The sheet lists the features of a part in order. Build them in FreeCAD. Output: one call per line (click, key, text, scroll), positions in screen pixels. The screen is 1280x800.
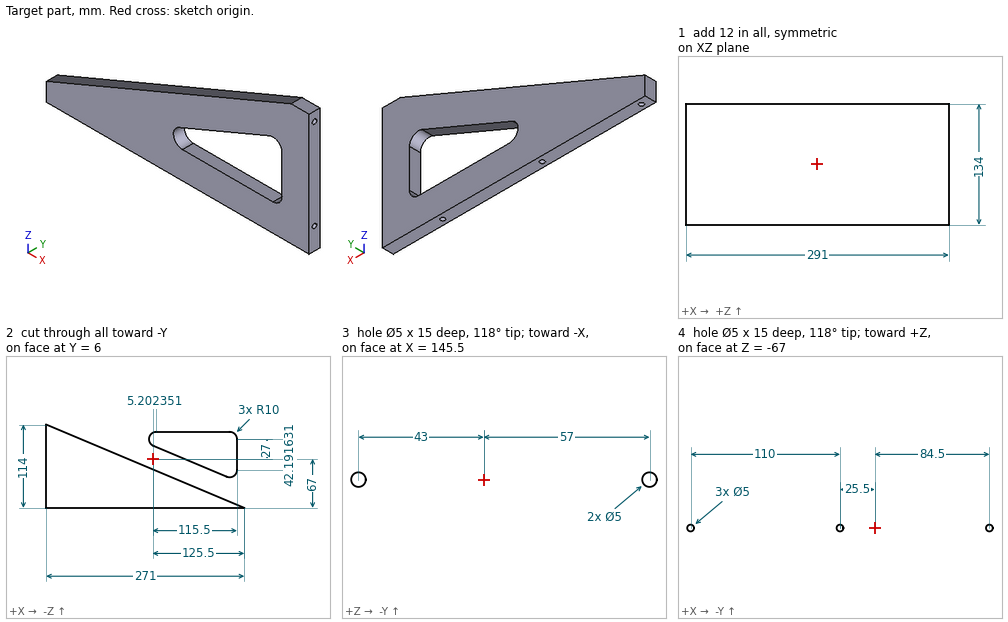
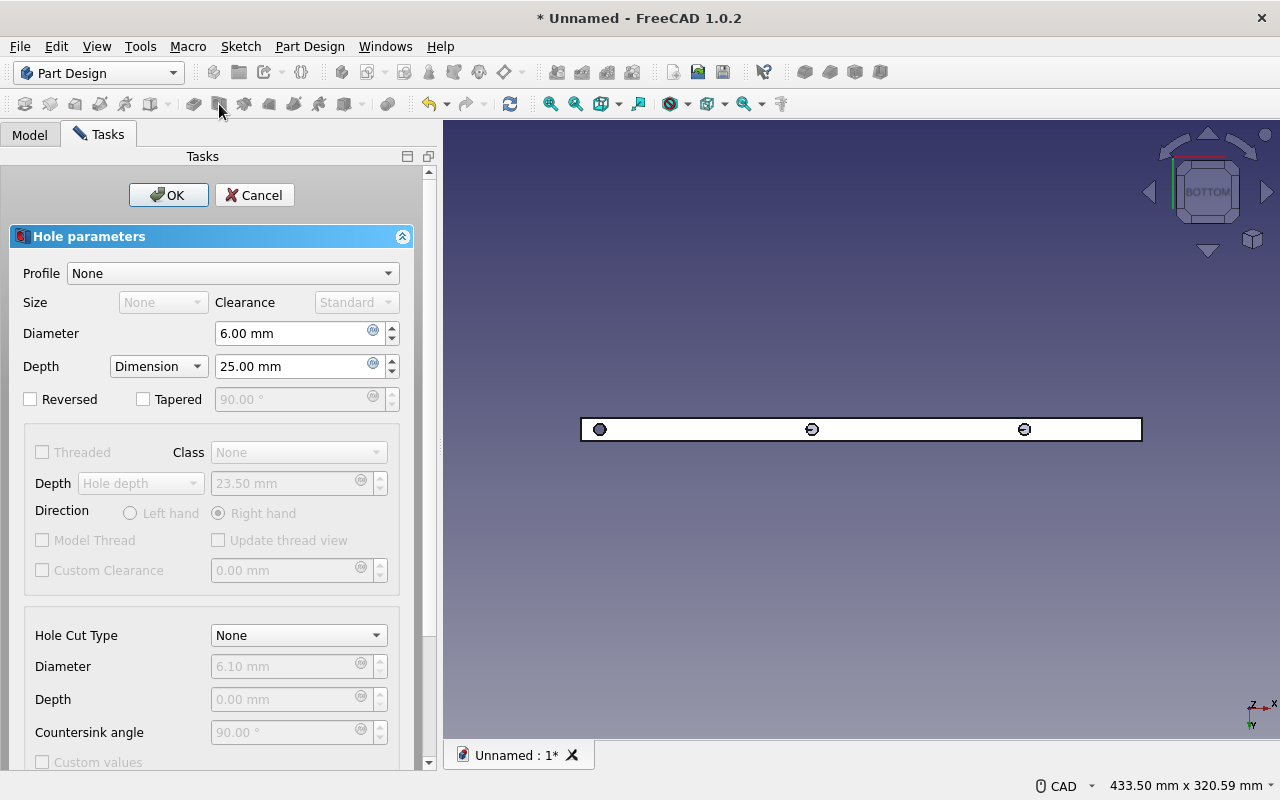
triple_click(300, 334)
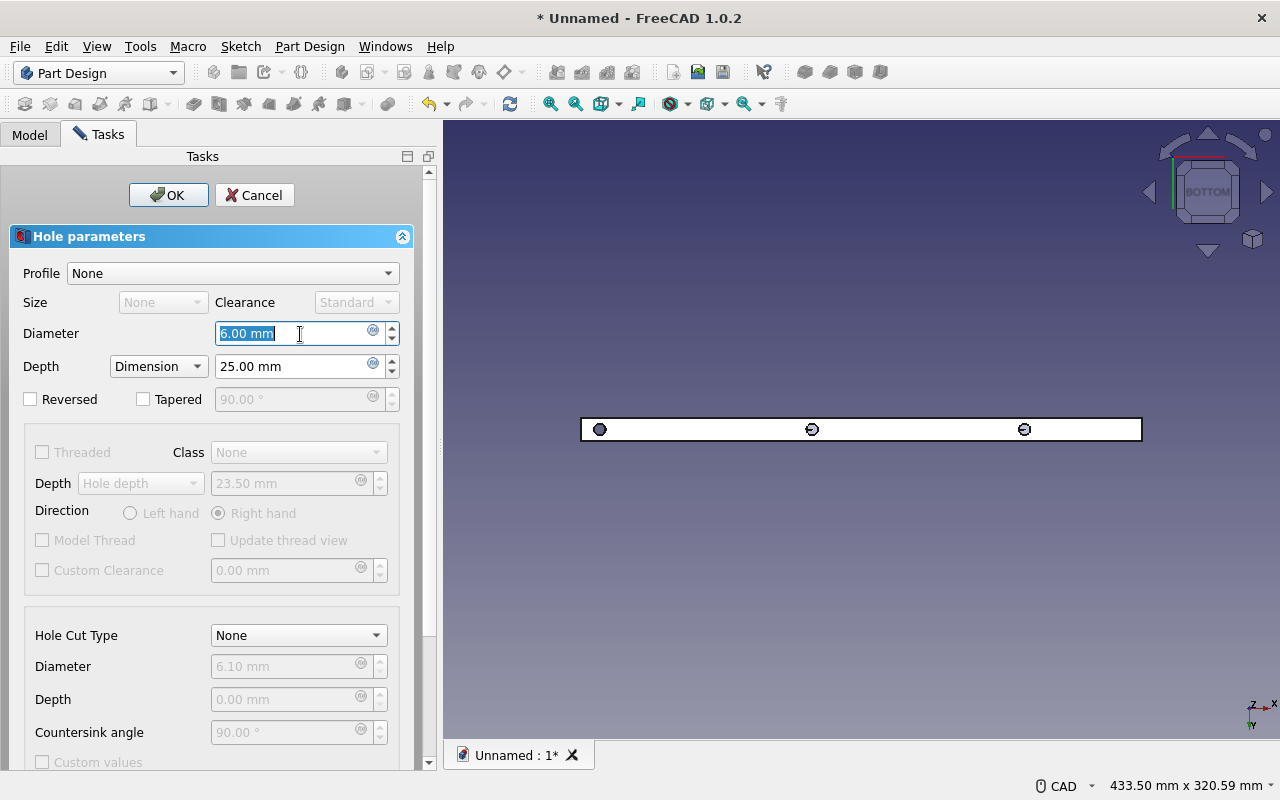
text(5)
key(Tab)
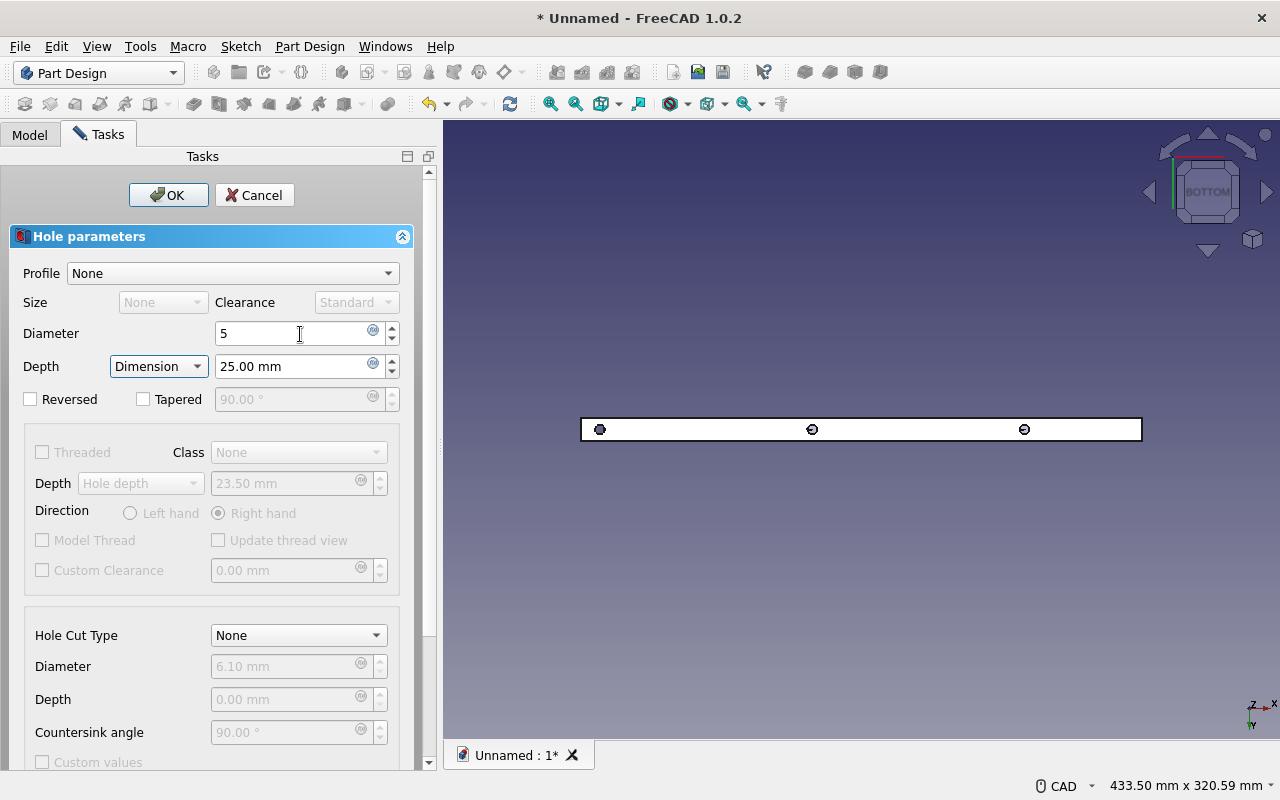
triple_click(300, 366)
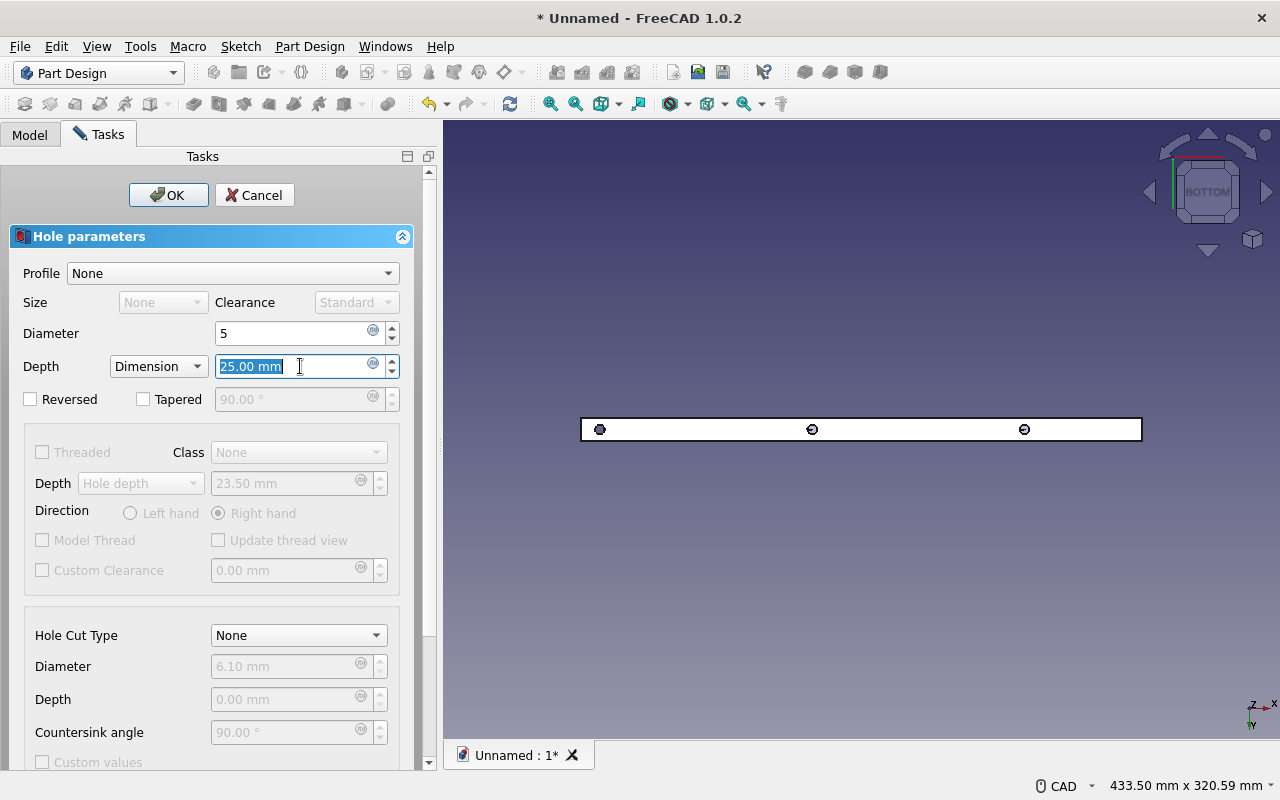
text(15)
key(Tab)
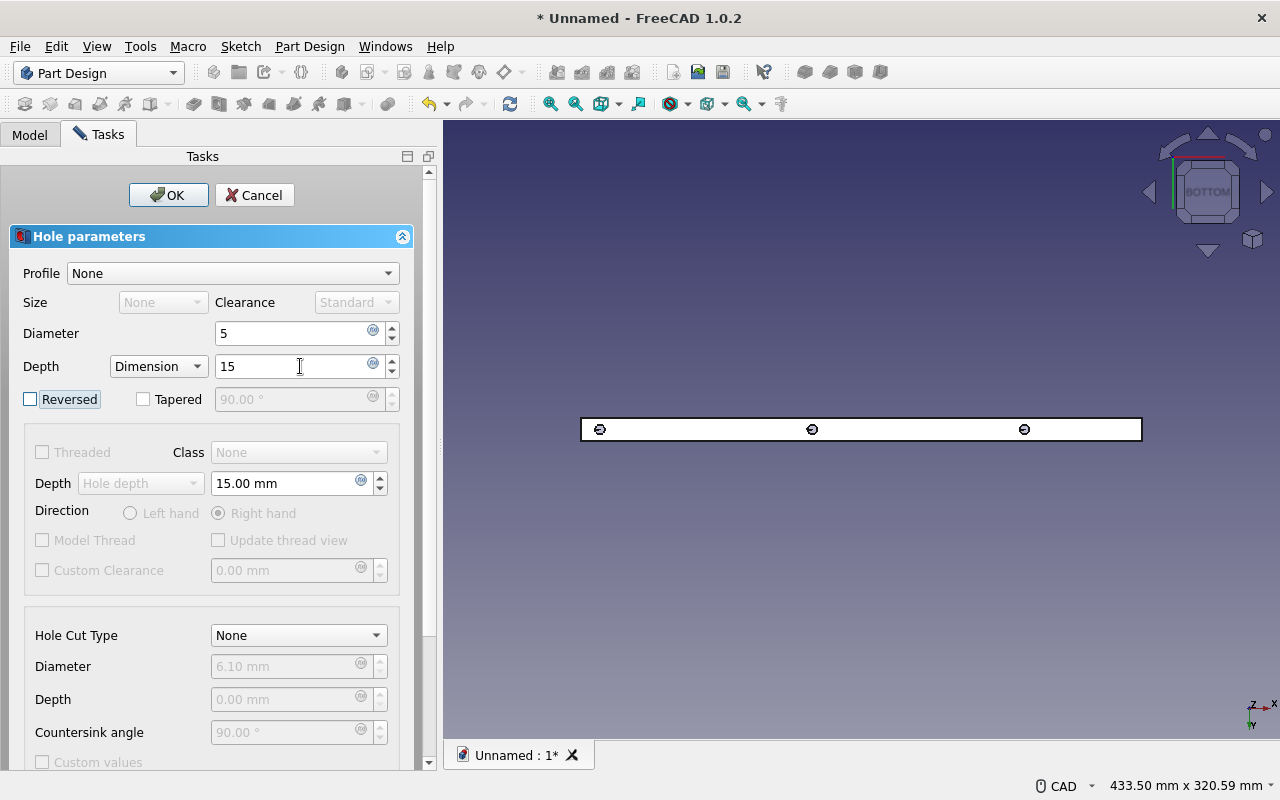
click(169, 195)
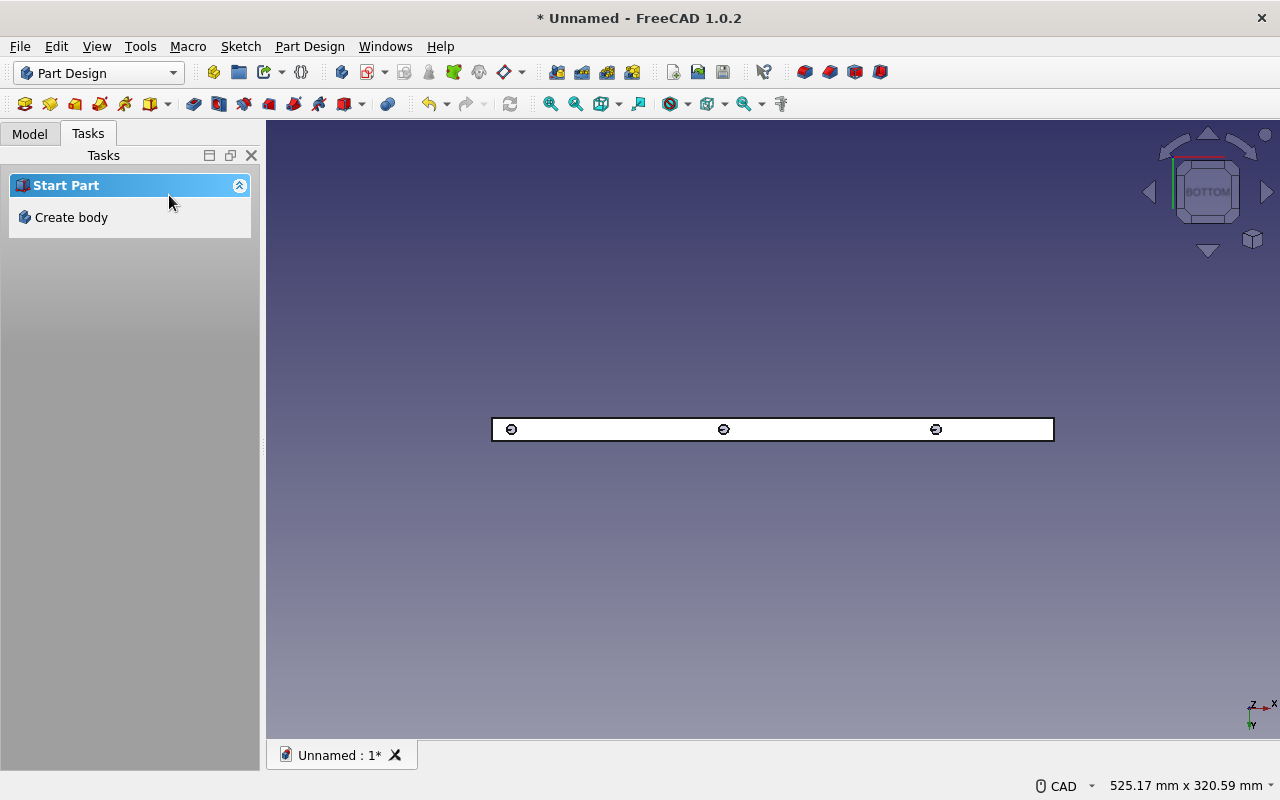
key(0)